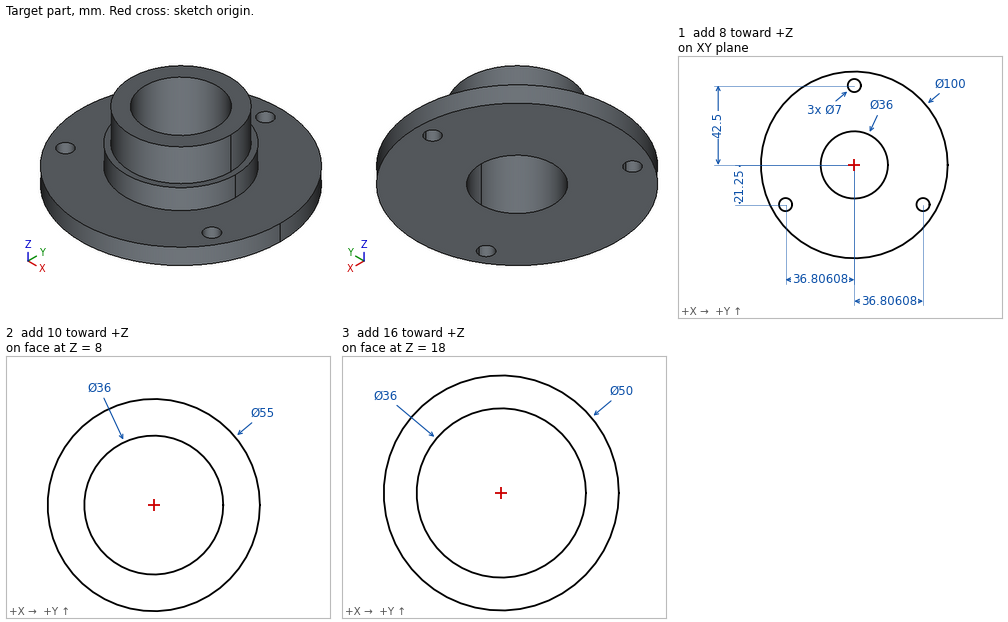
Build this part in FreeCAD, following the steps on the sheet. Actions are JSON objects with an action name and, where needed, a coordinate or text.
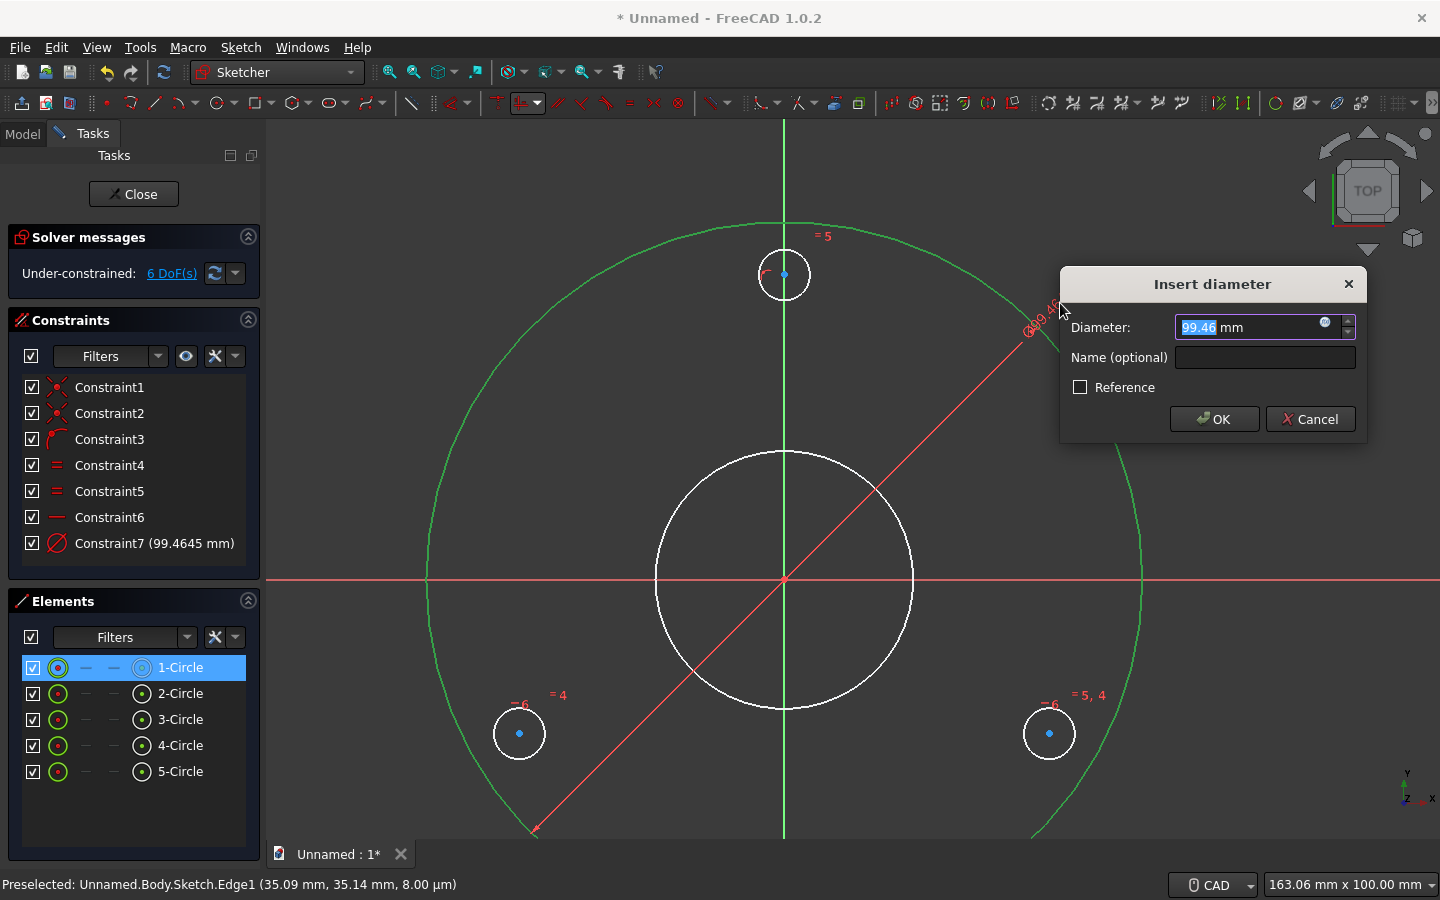
{"action": "type", "text": "100"}
{"action": "key", "text": "Return"}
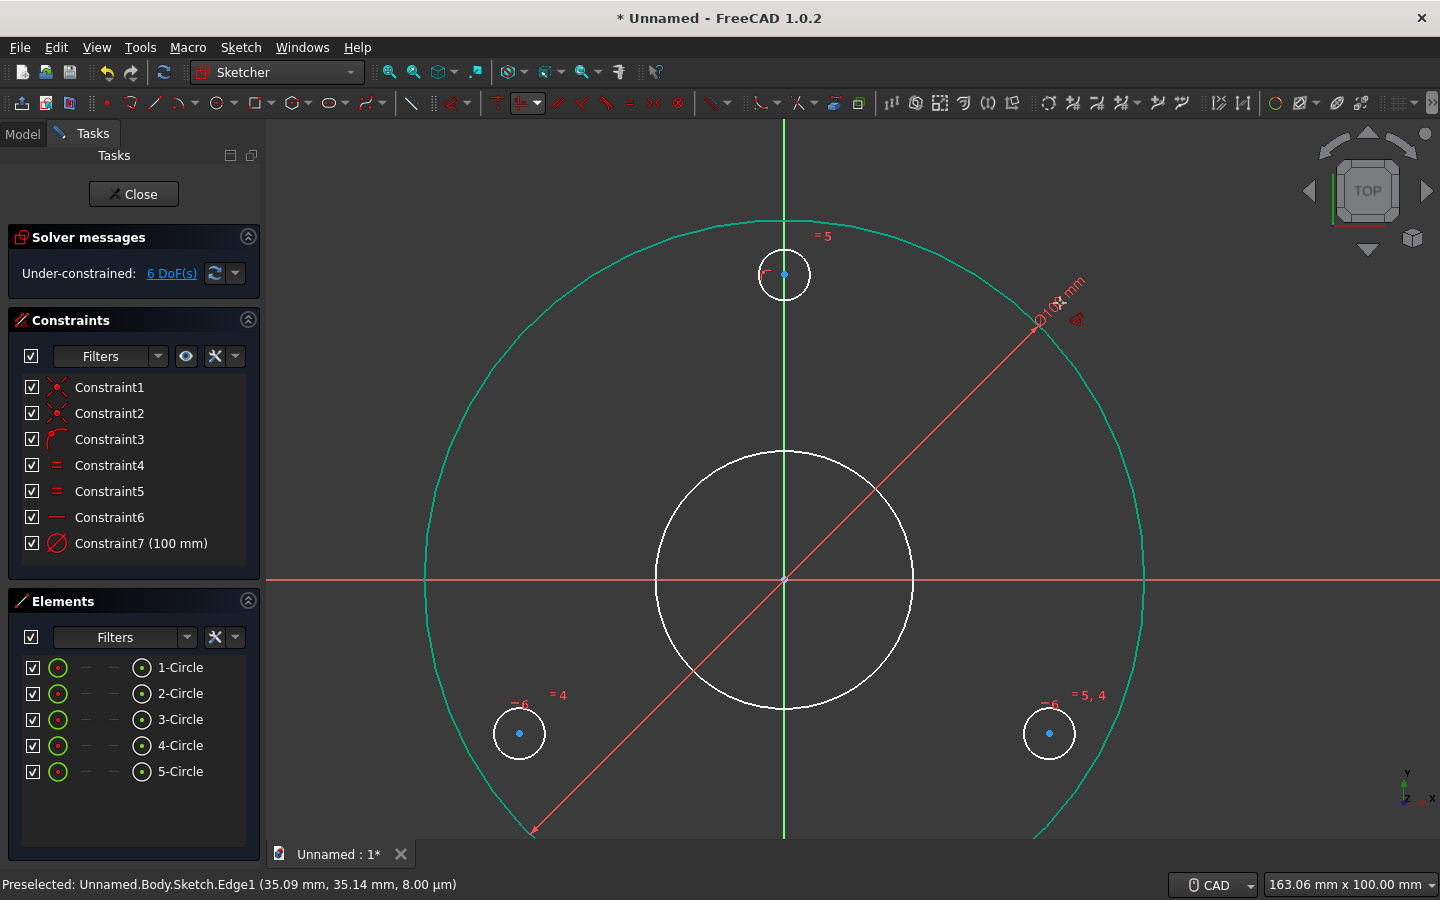
{"action": "left_click", "coordinate": [537, 716]}
{"action": "left_click", "coordinate": [560, 693]}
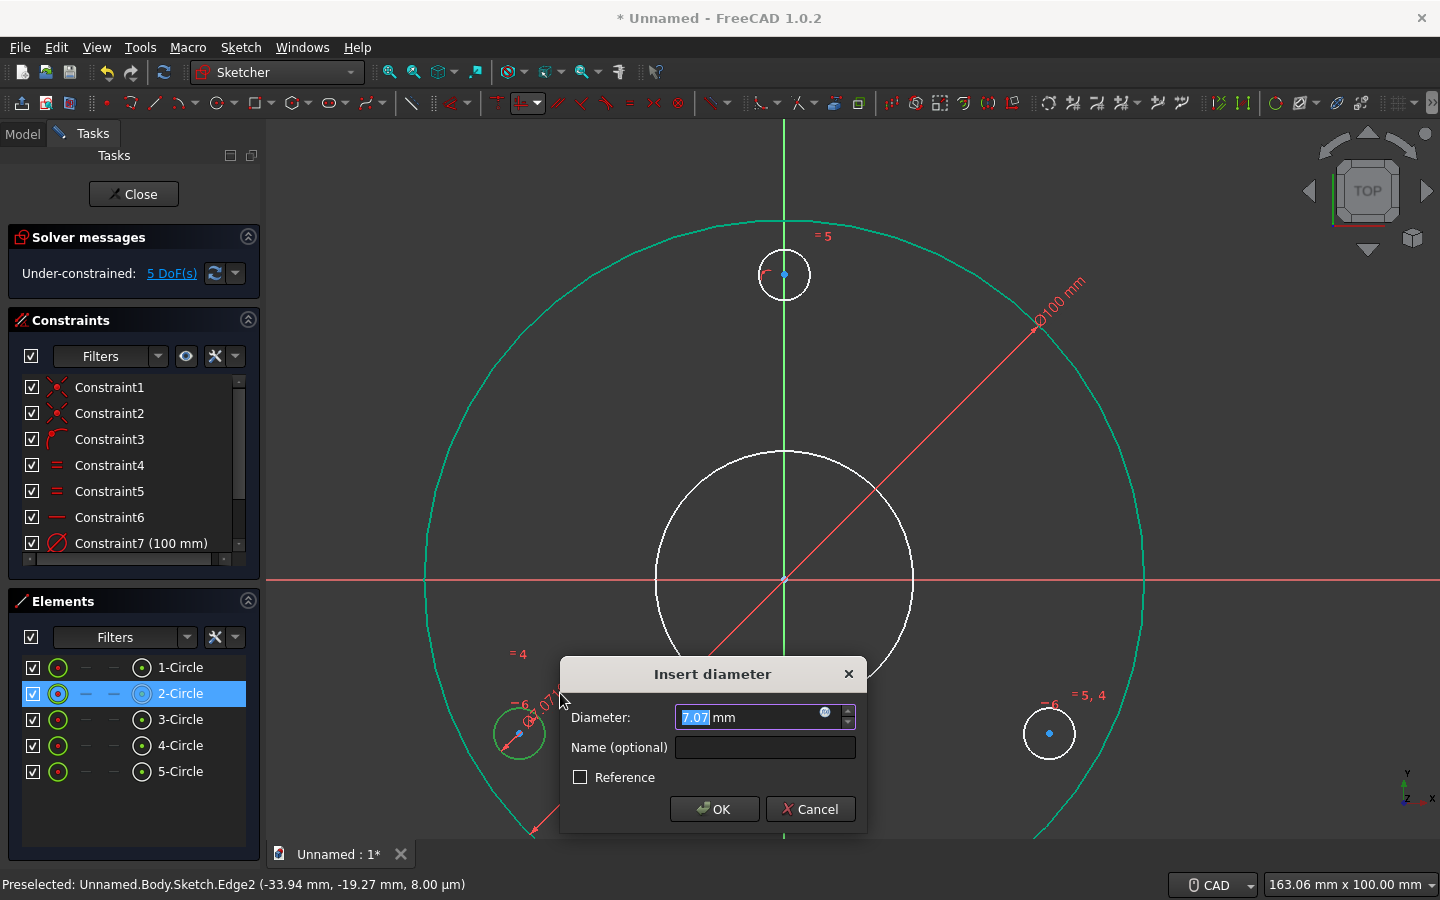
{"action": "type", "text": "7"}
{"action": "key", "text": "Return"}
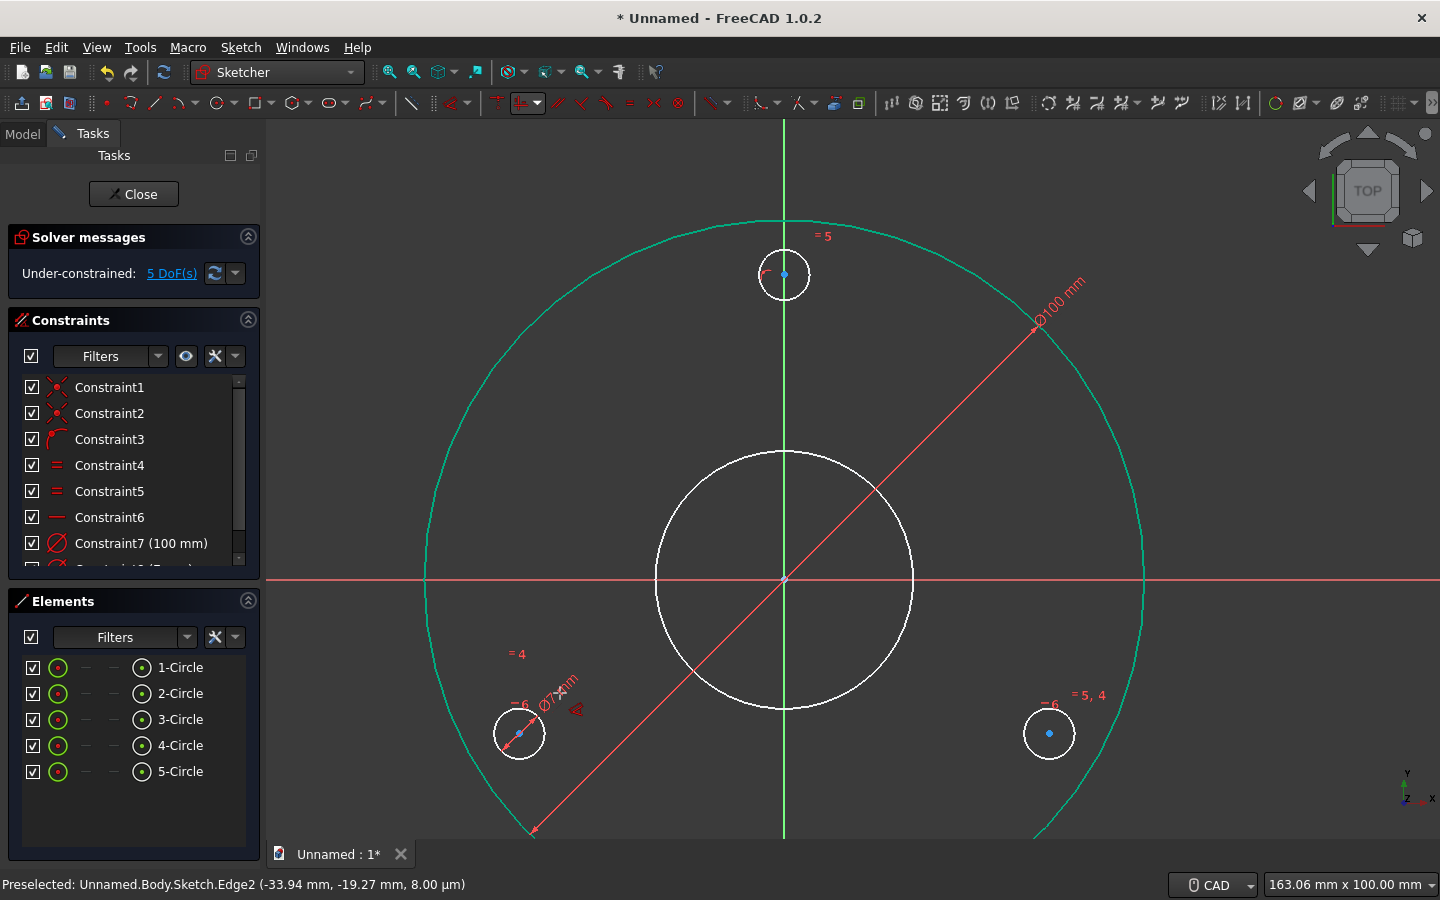
{"action": "left_click", "coordinate": [875, 489]}
{"action": "left_click", "coordinate": [898, 466]}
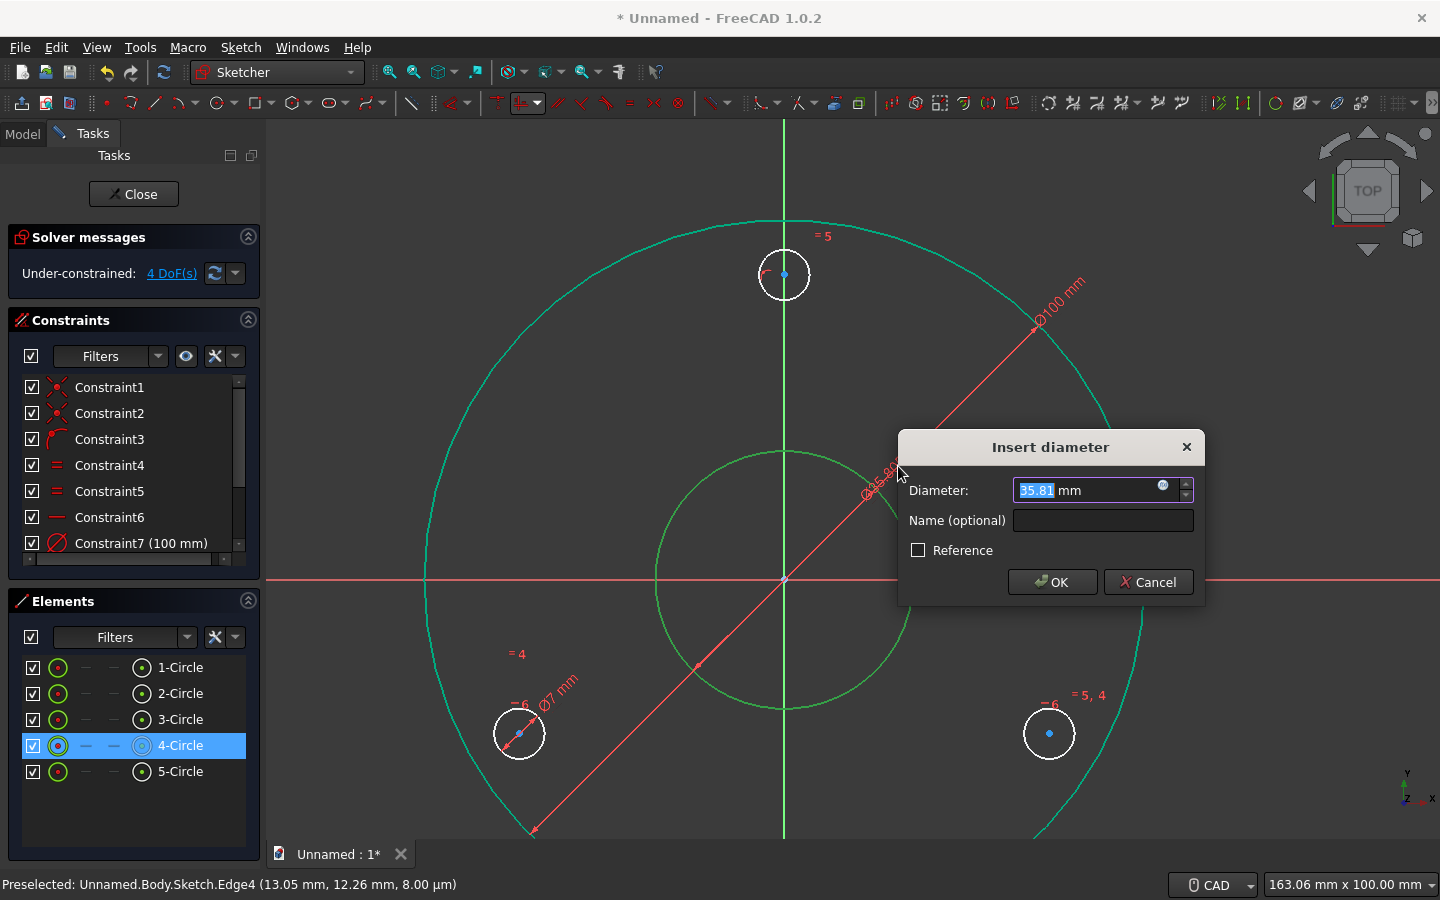
{"action": "type", "text": "36"}
{"action": "key", "text": "Return"}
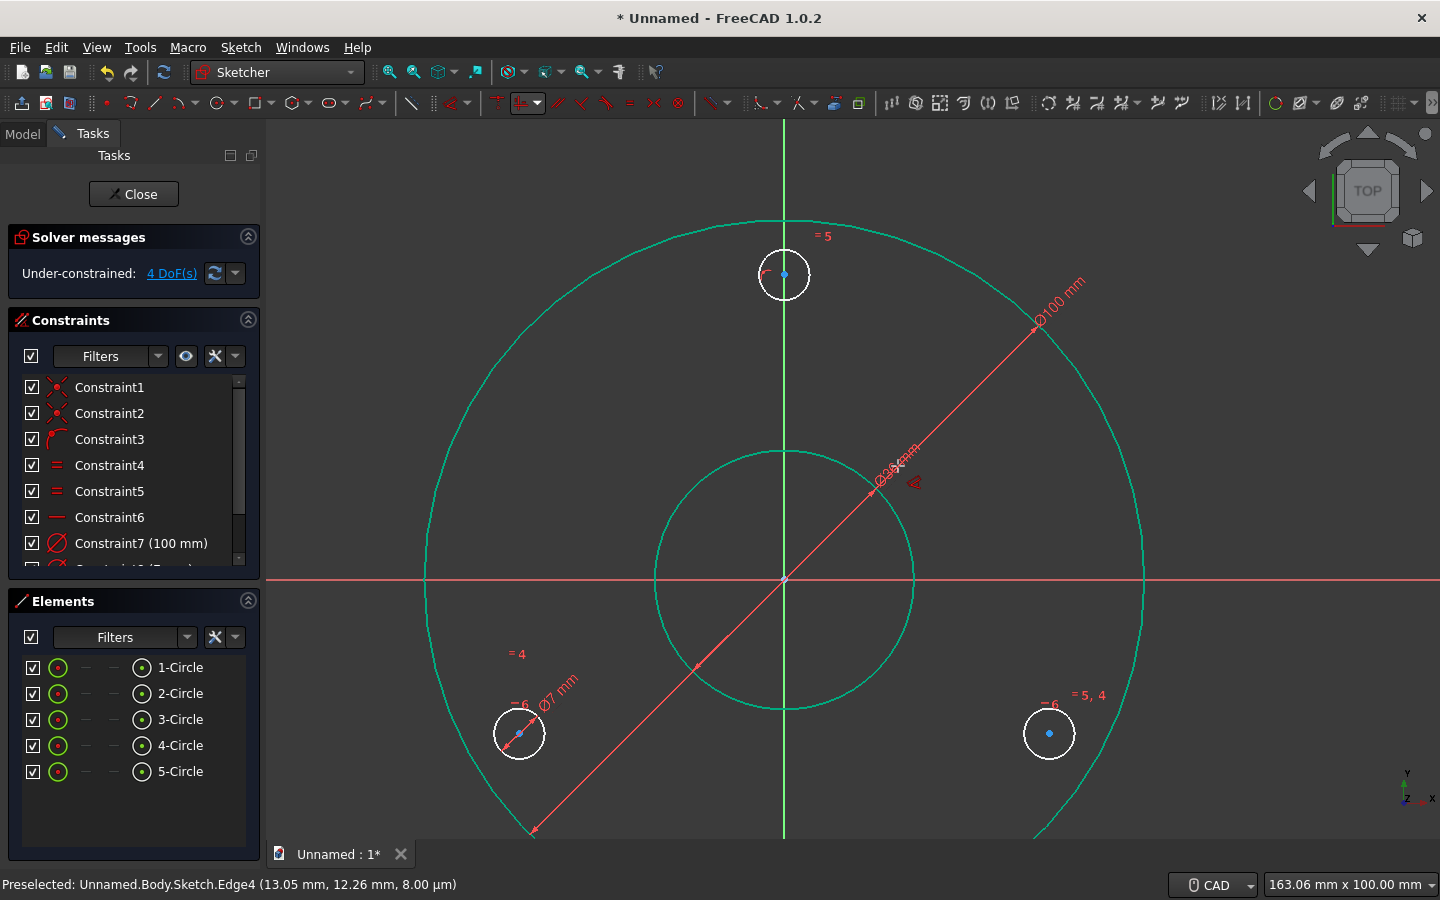
{"action": "left_click", "coordinate": [784, 275]}
{"action": "left_click", "coordinate": [818, 427]}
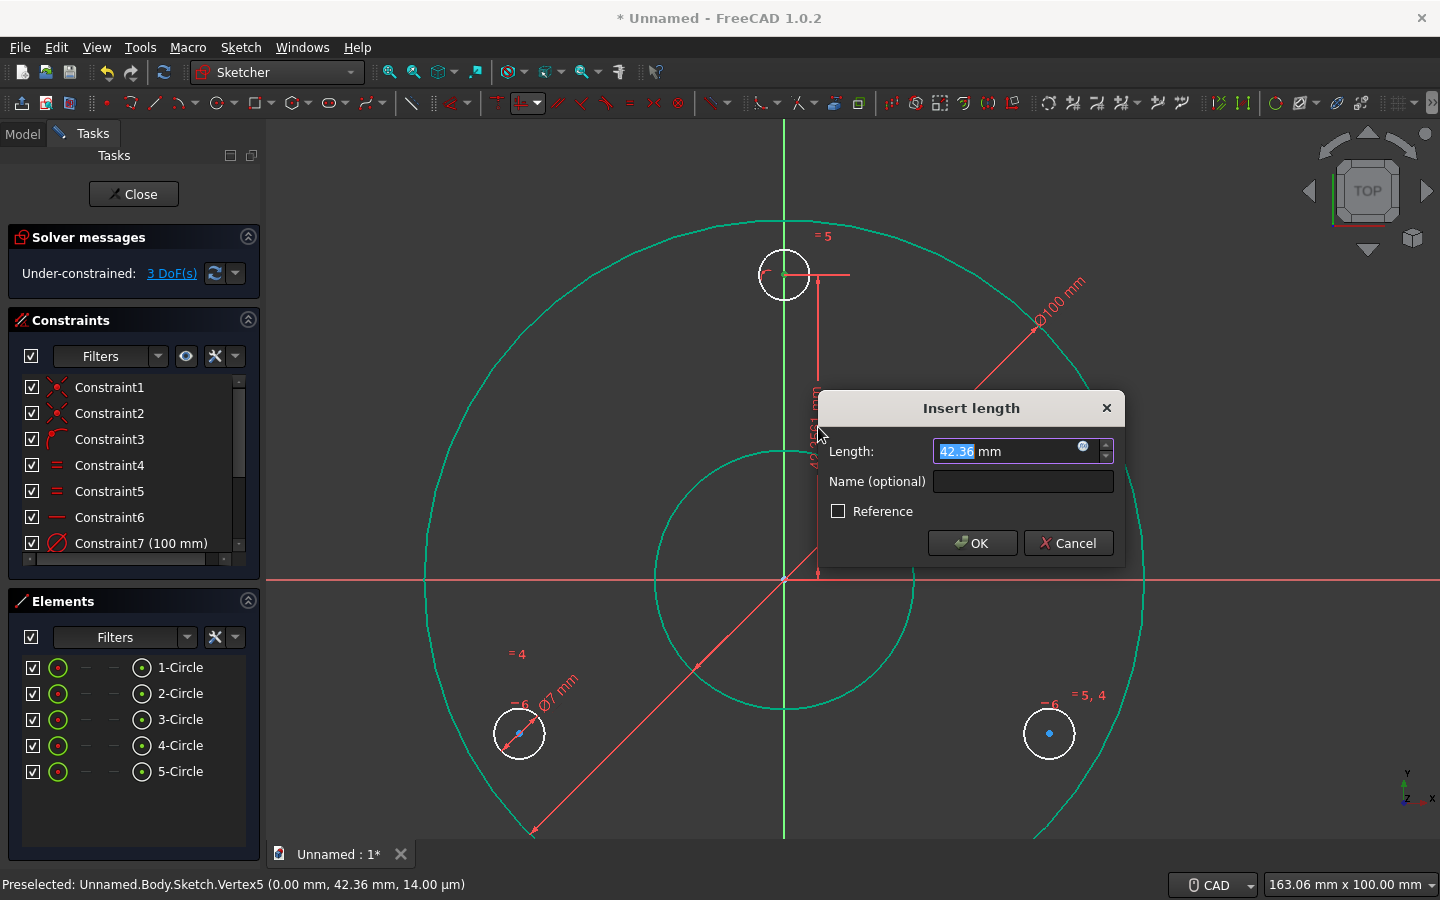
{"action": "type", "text": "42.5"}
{"action": "key", "text": "Return"}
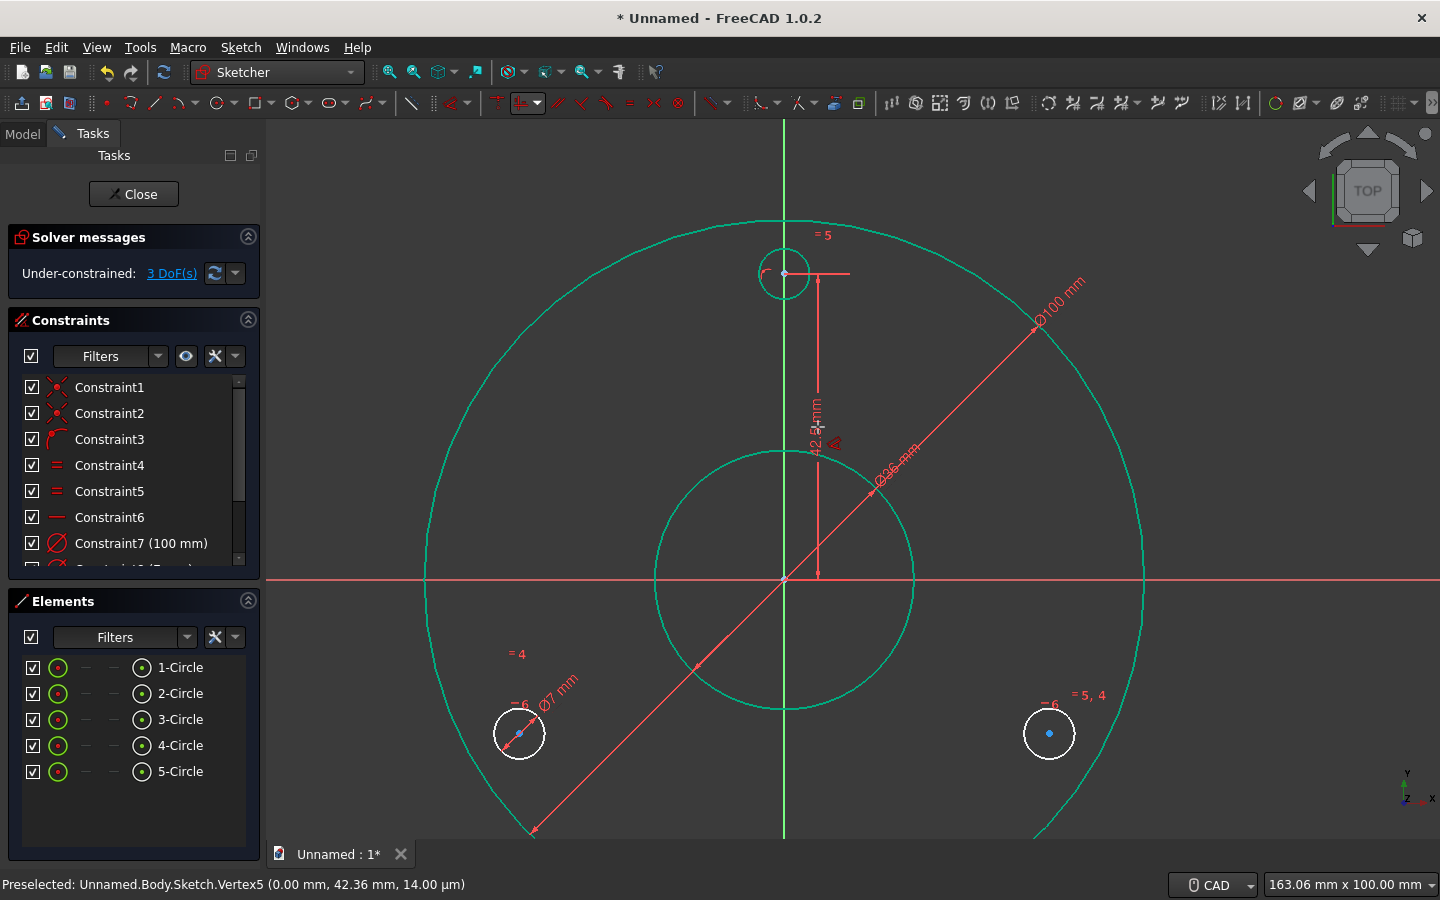
{"action": "left_click", "coordinate": [519, 734]}
{"action": "left_click", "coordinate": [485, 657]}